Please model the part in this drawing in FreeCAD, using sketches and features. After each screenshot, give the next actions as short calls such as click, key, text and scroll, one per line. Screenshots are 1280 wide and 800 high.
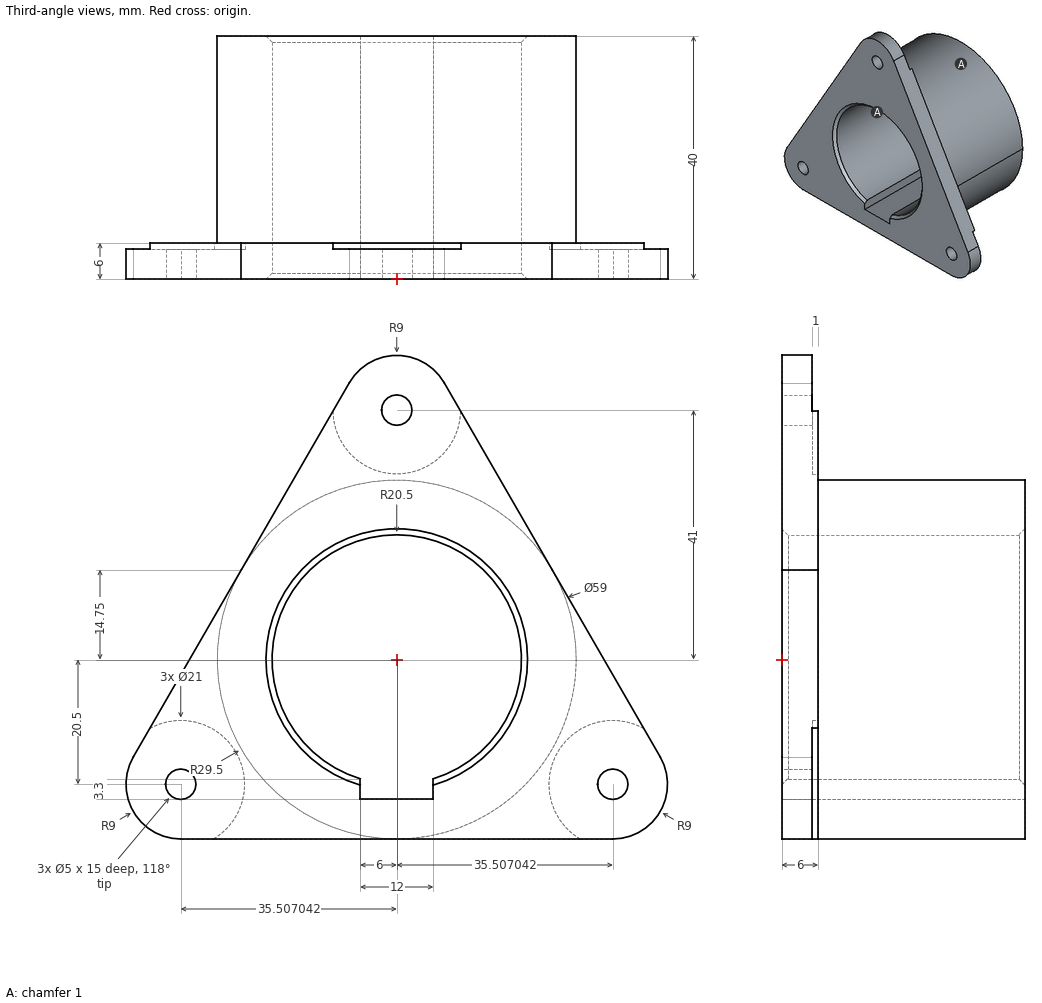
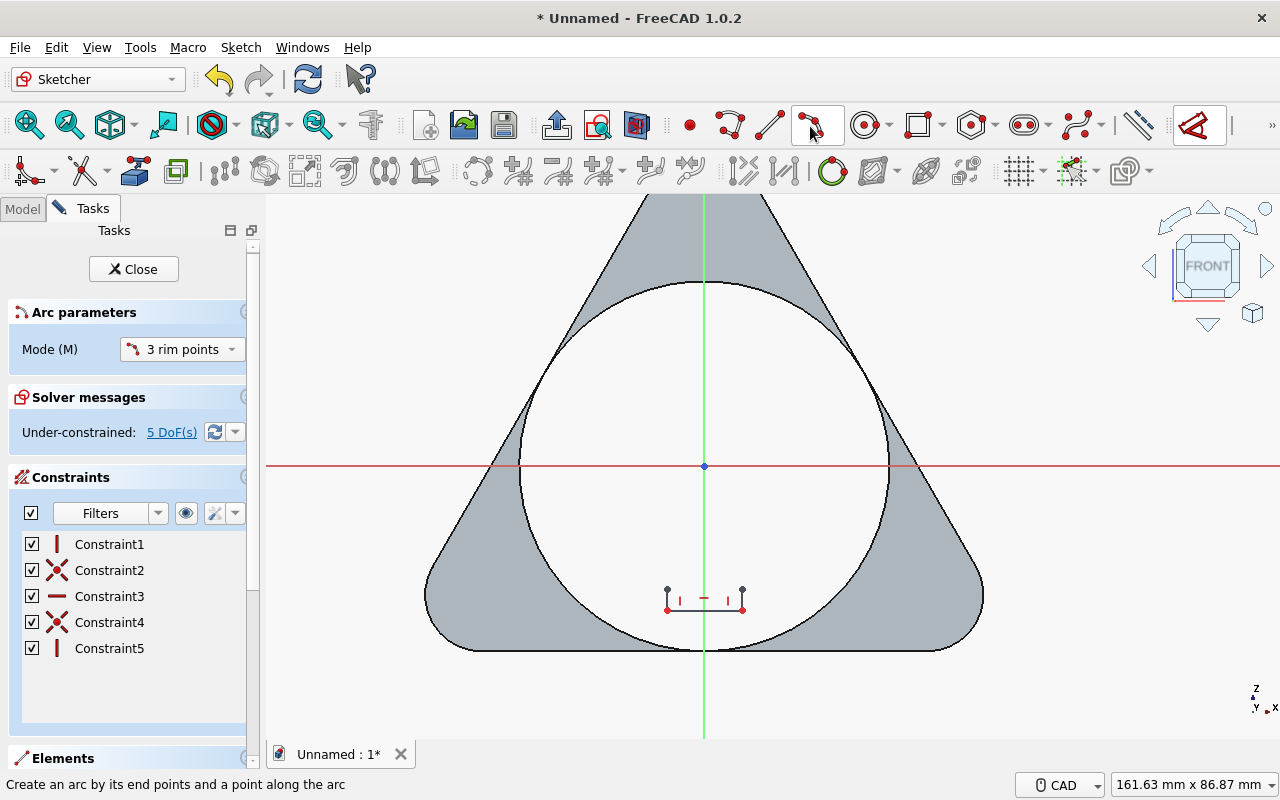
scroll(742, 589, up, 3)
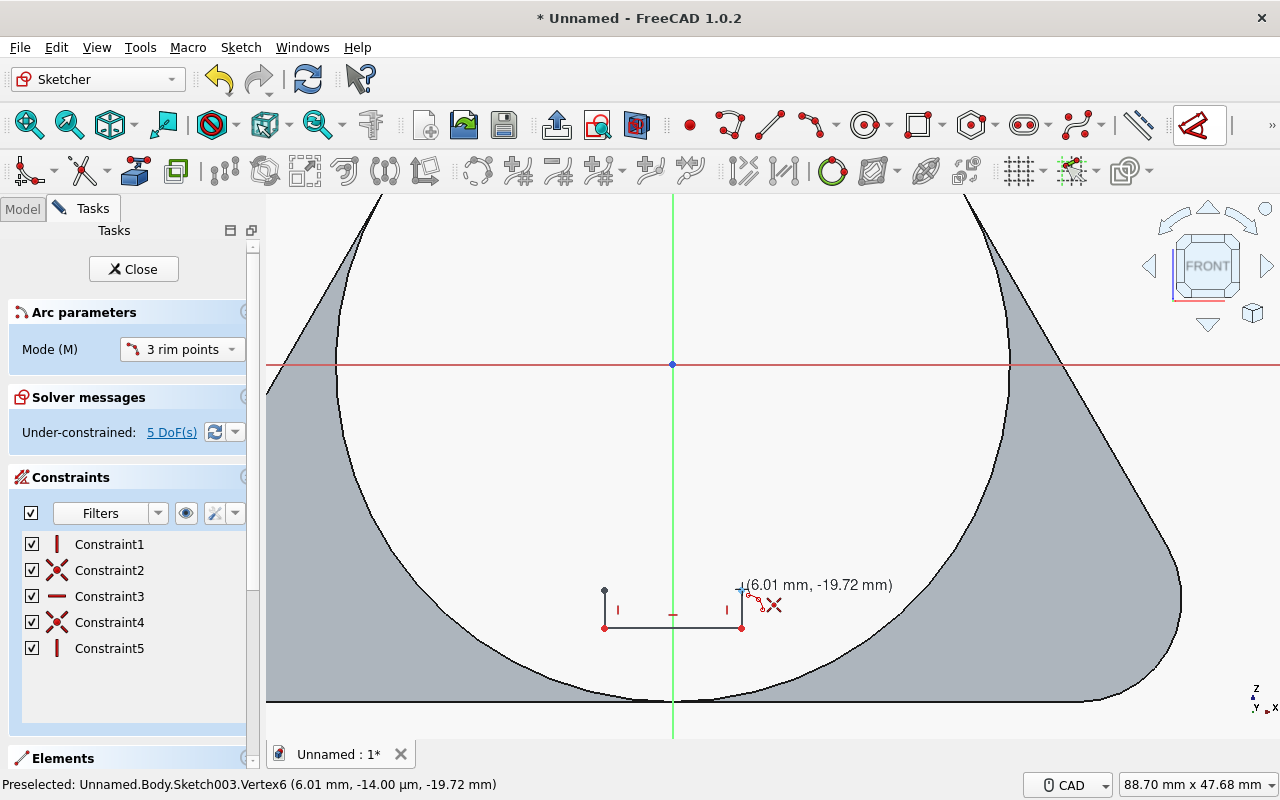
click(742, 590)
click(605, 590)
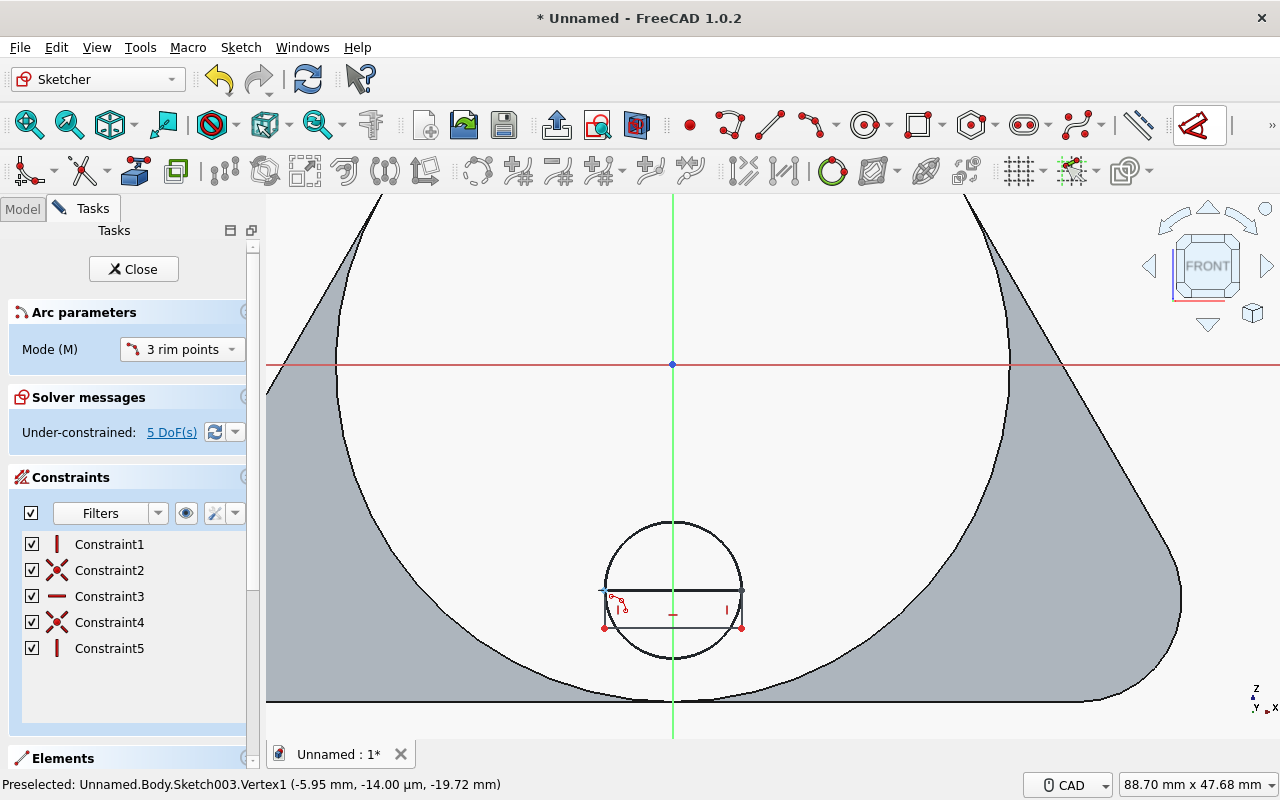
scroll(743, 590, down, 3)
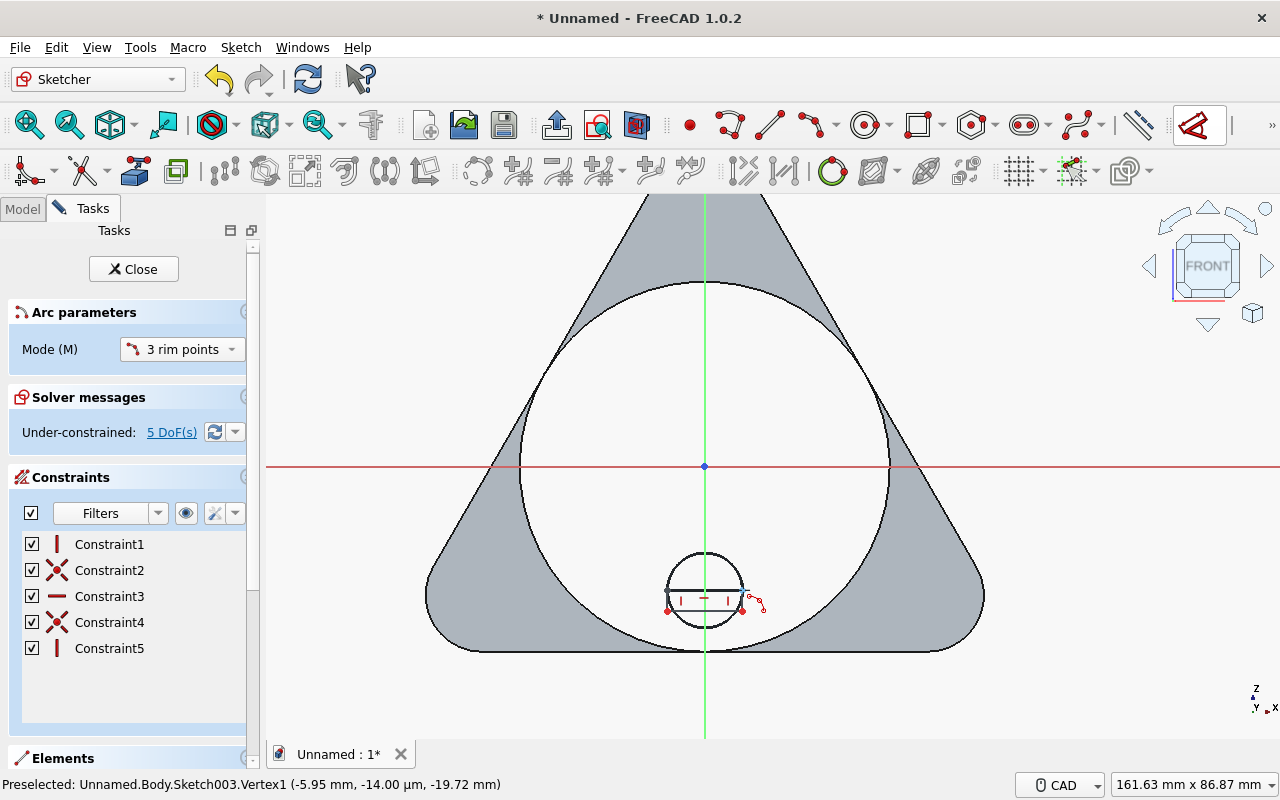
click(774, 358)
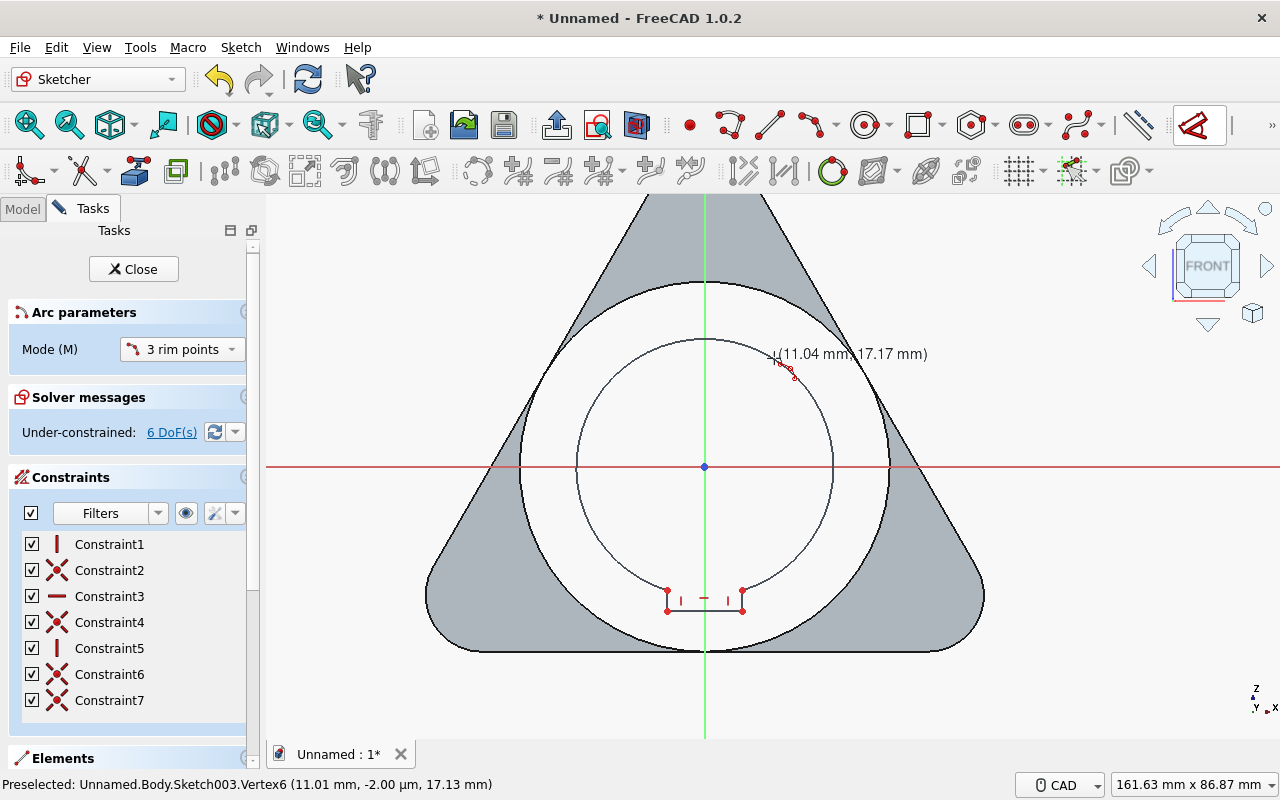
click(866, 126)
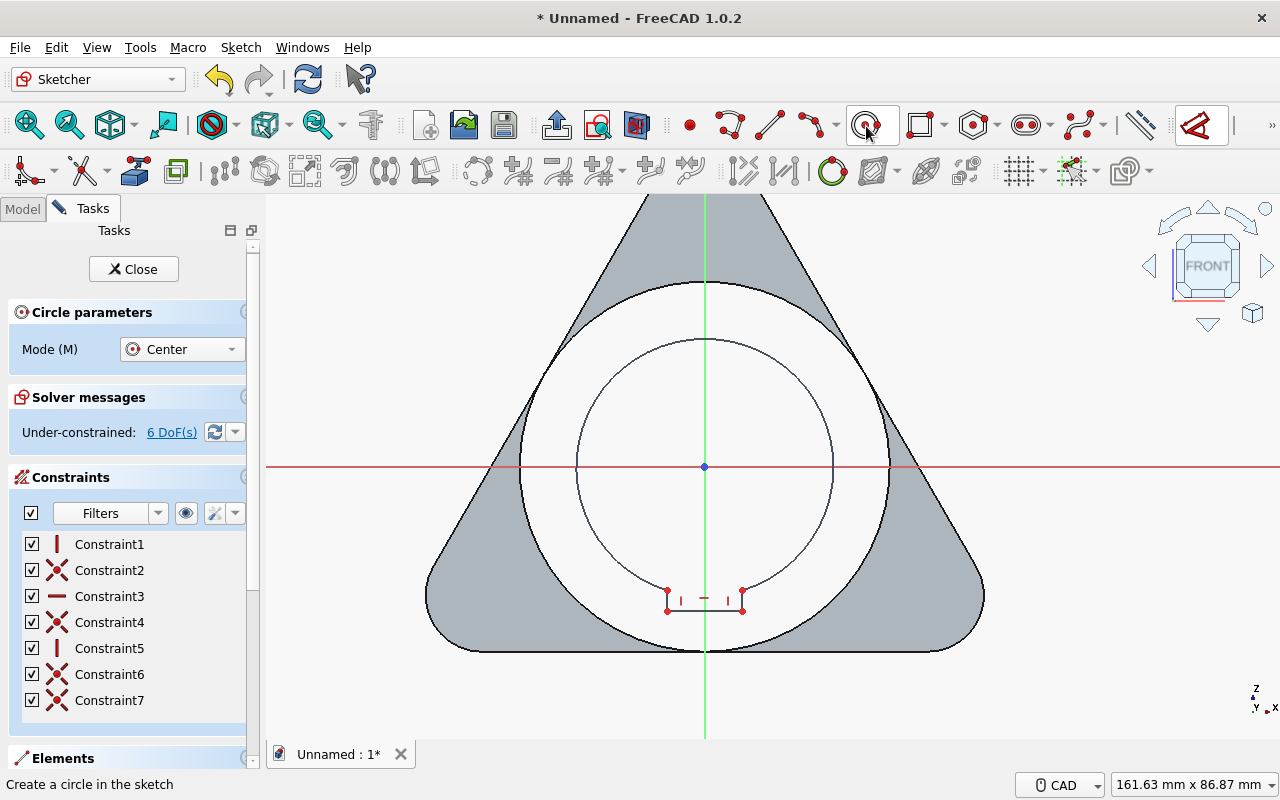
click(705, 467)
click(836, 336)
key(Escape)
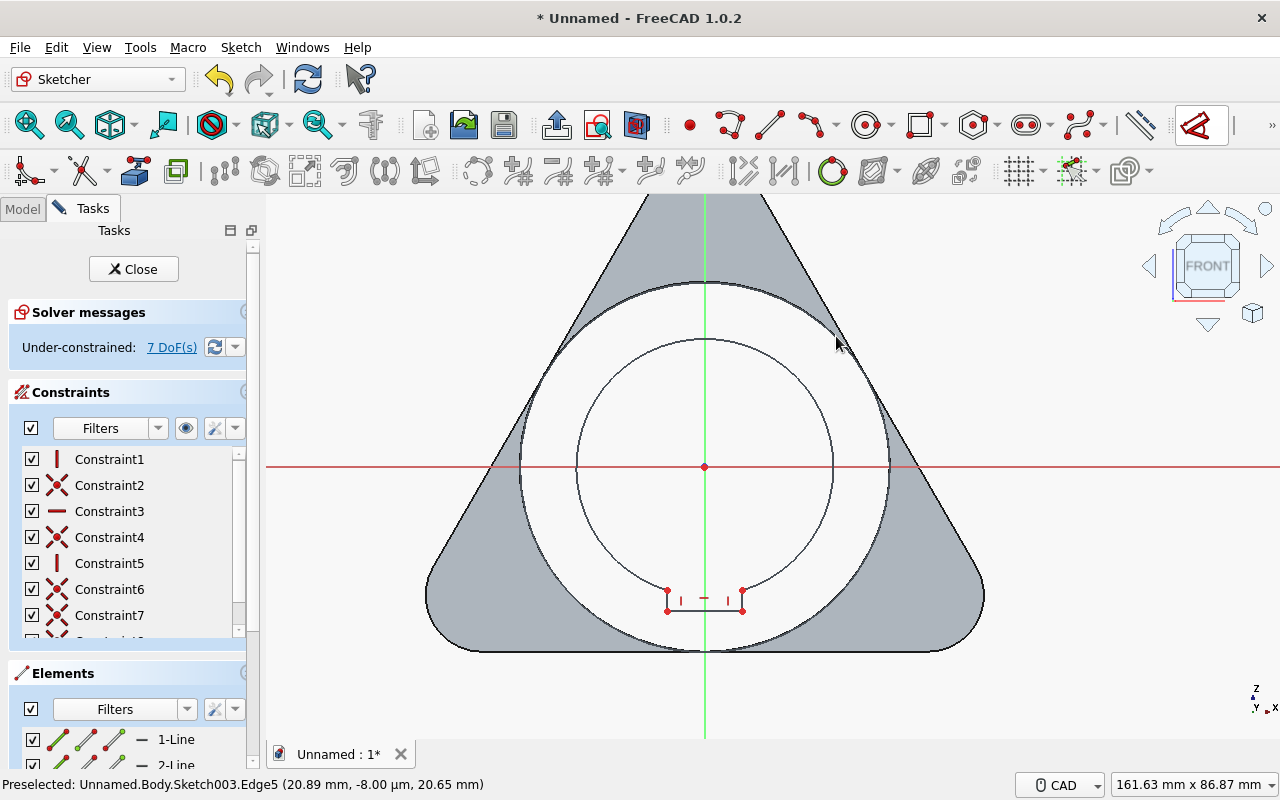
drag(695, 457, 715, 477)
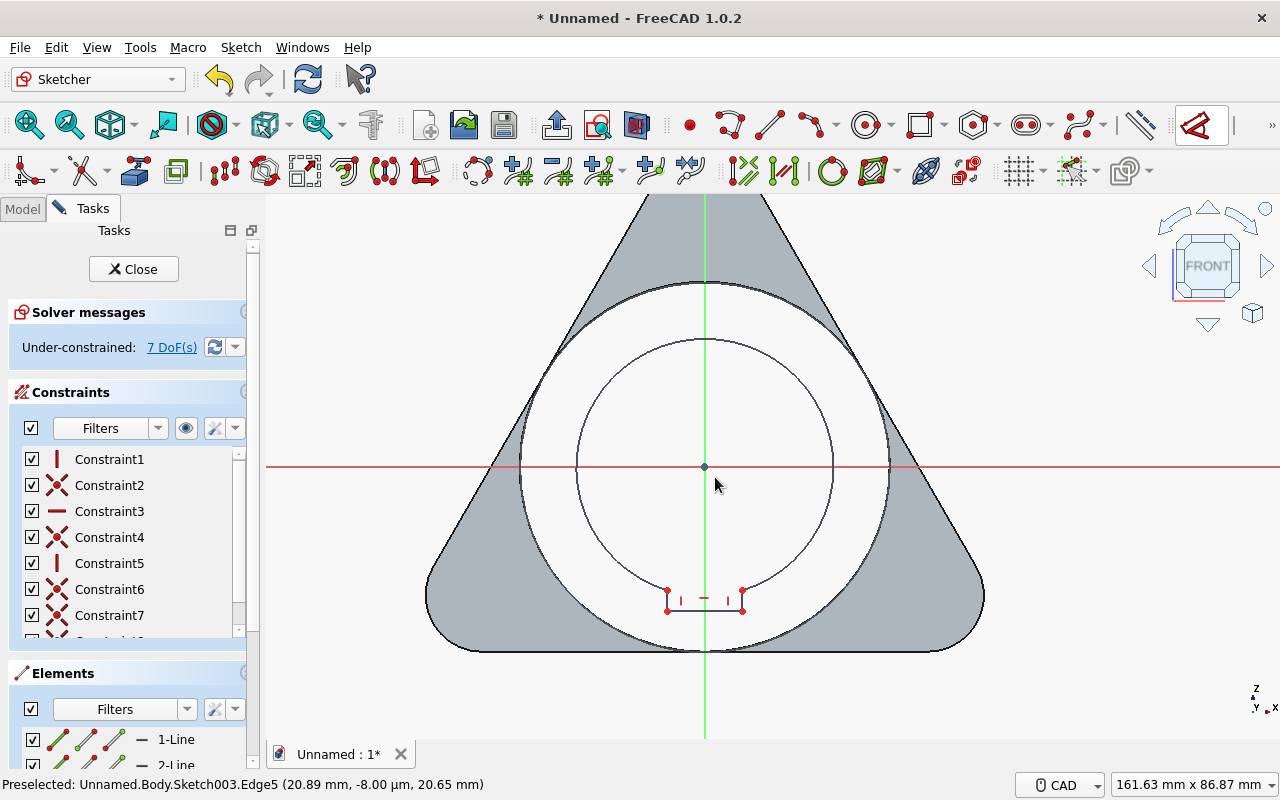
key(c)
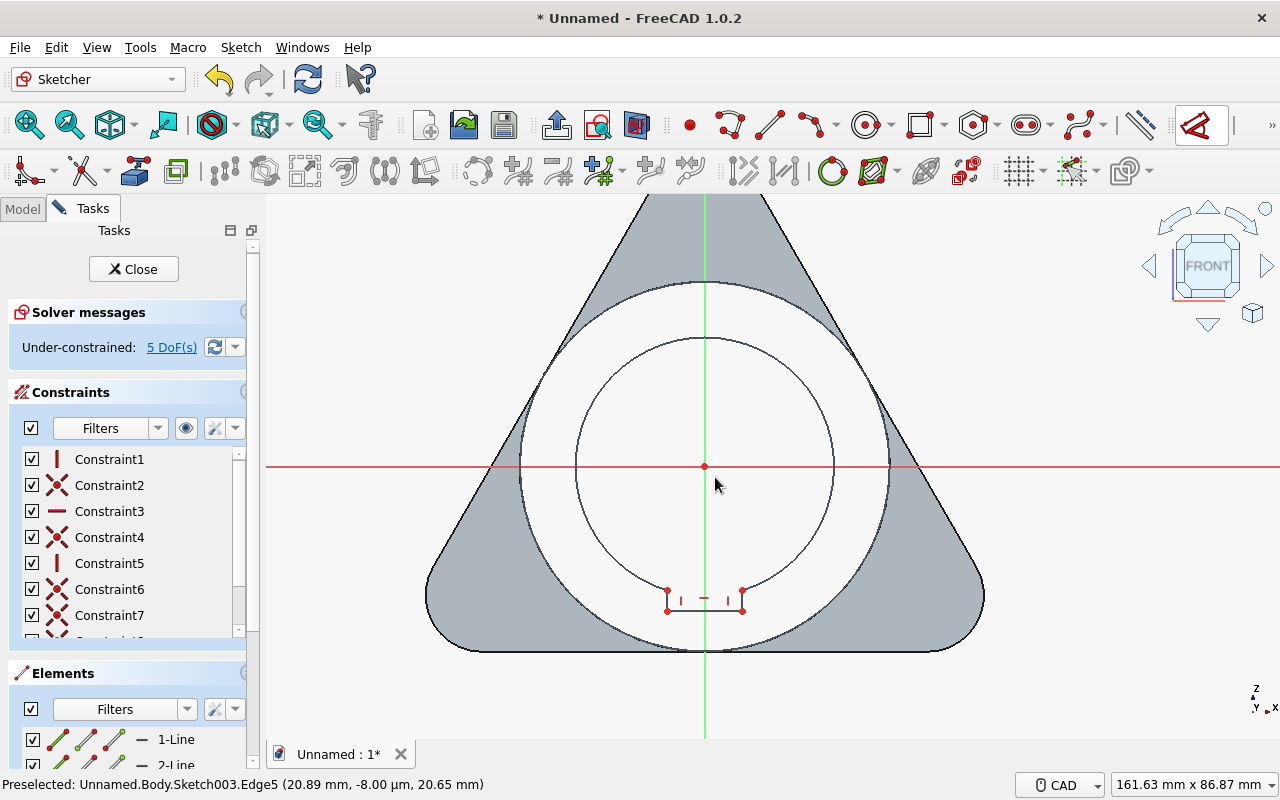
click(822, 412)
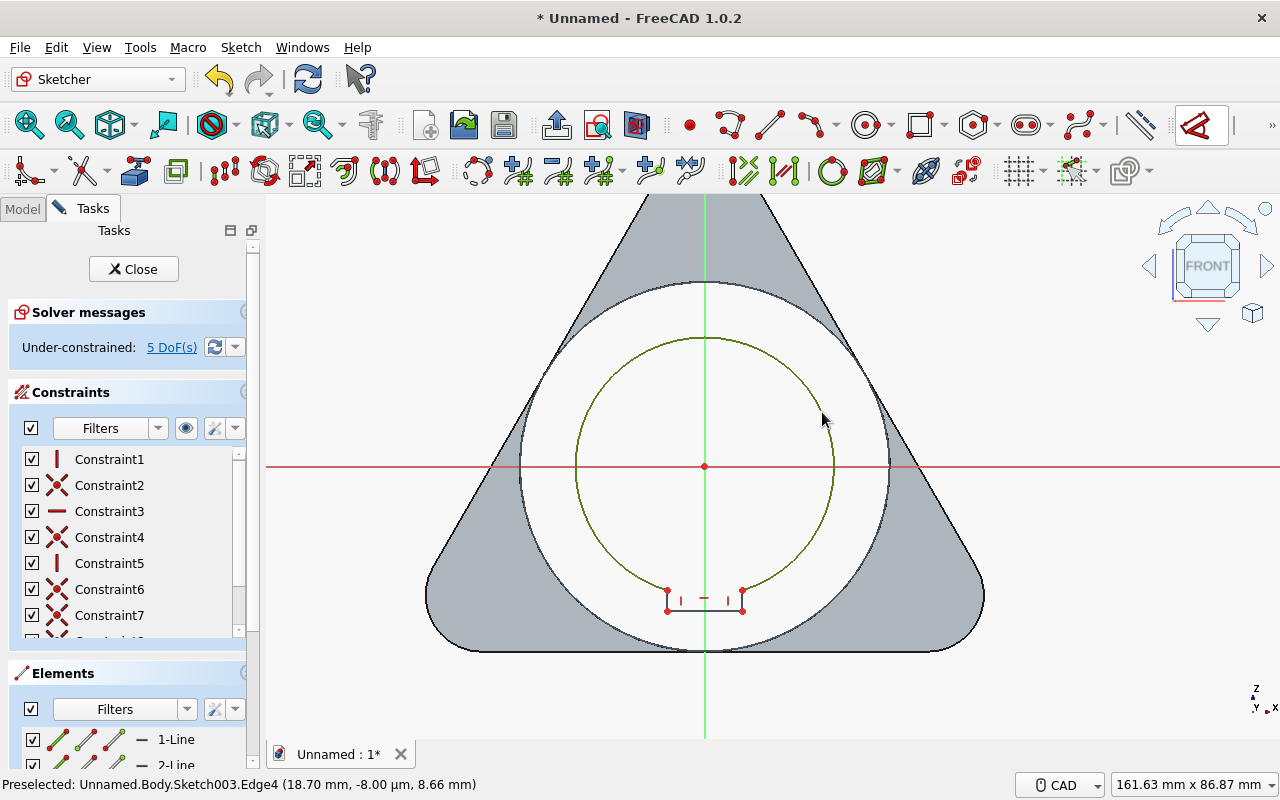
click(1222, 126)